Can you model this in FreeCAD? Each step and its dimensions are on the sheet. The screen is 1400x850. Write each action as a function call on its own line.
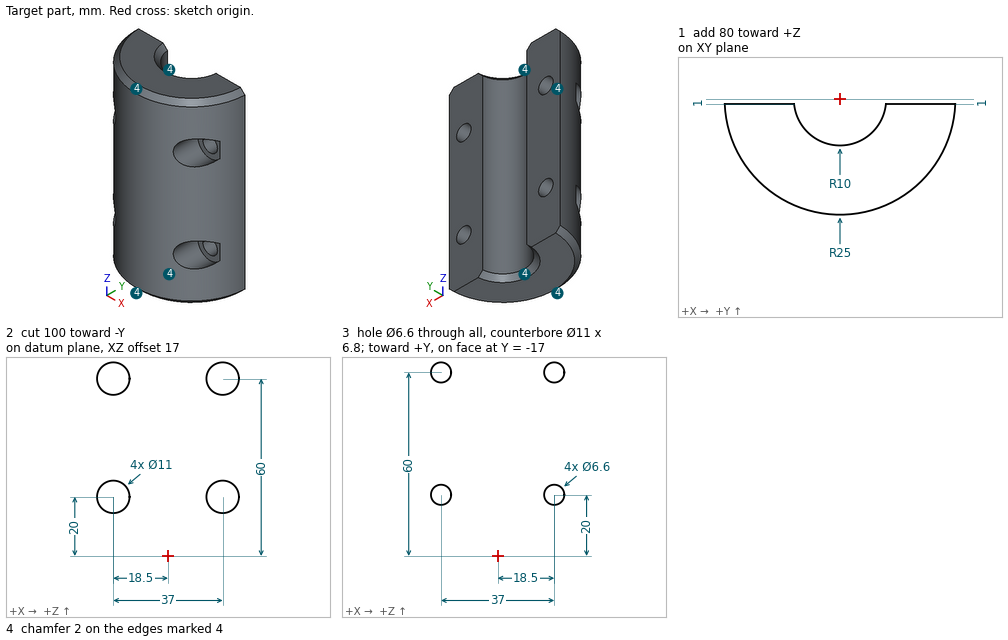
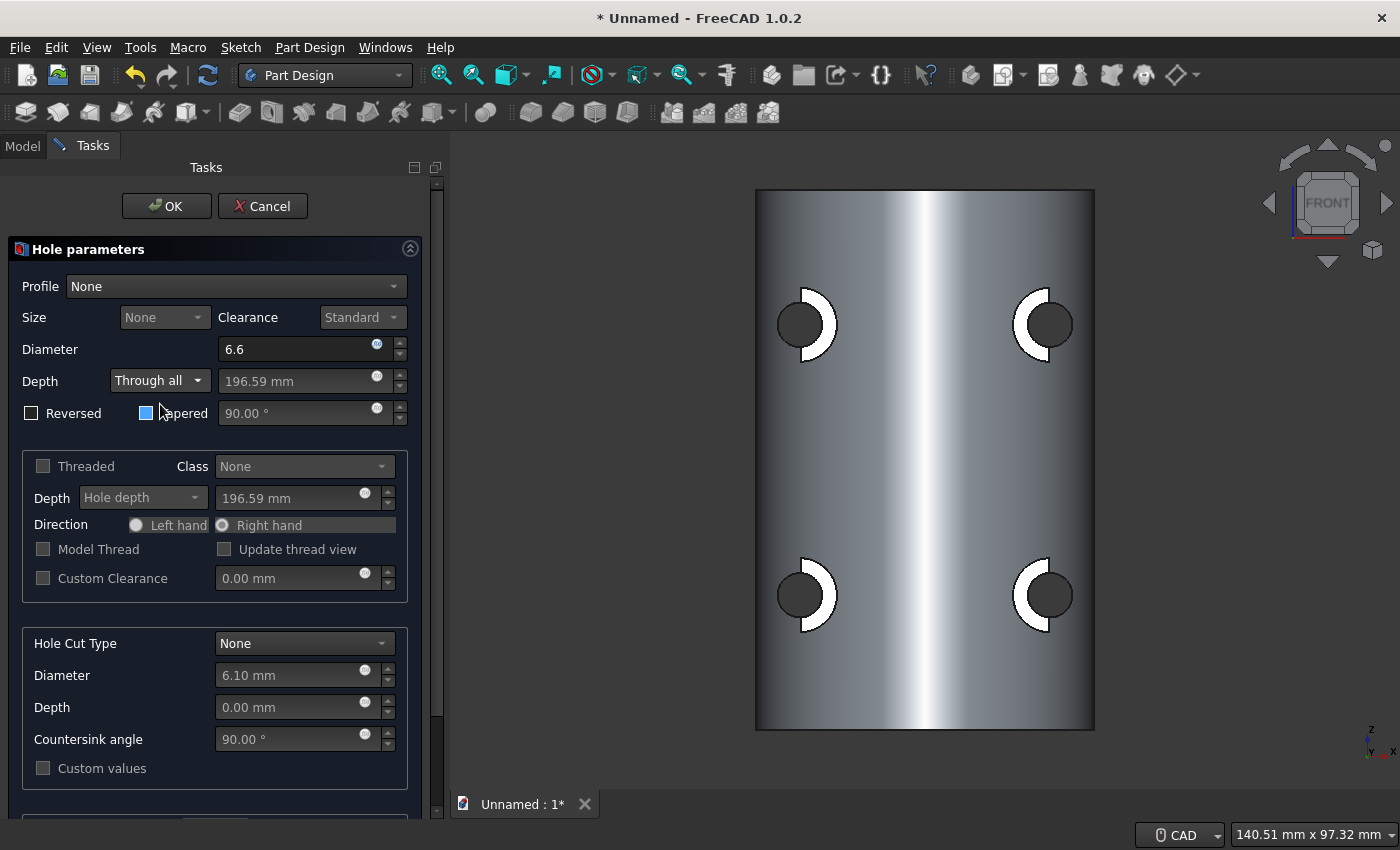
click(306, 644)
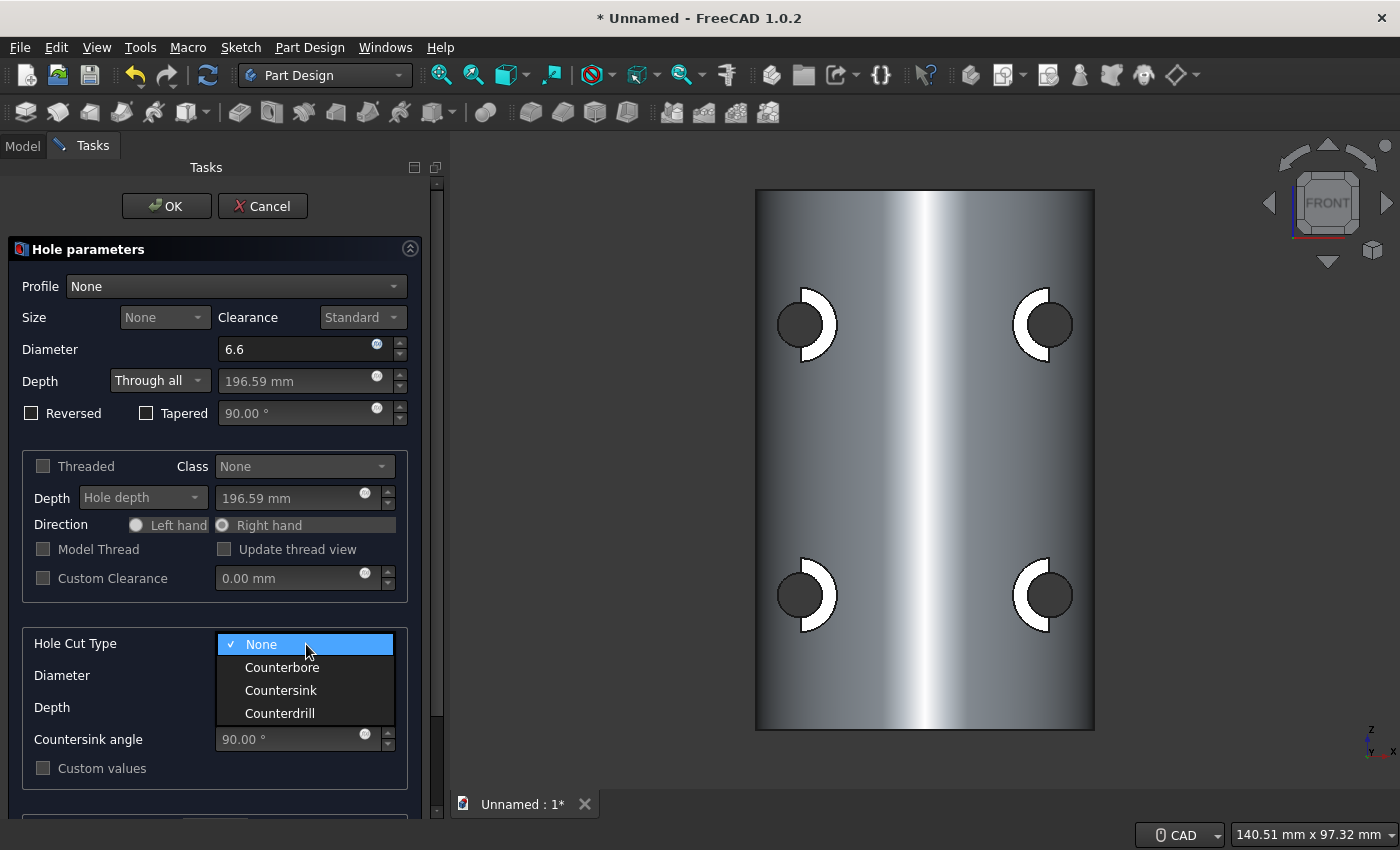
click(304, 668)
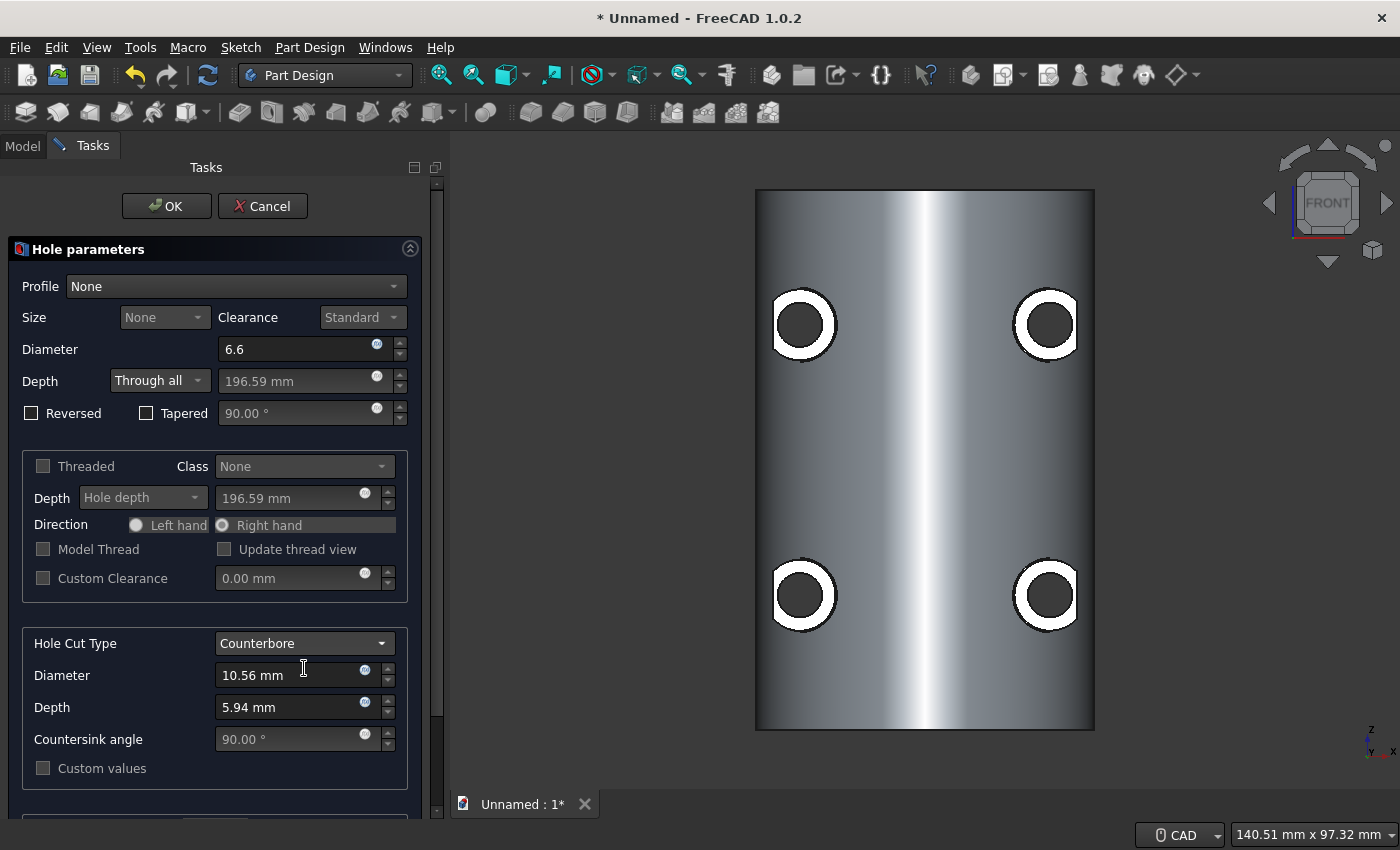
triple_click(298, 675)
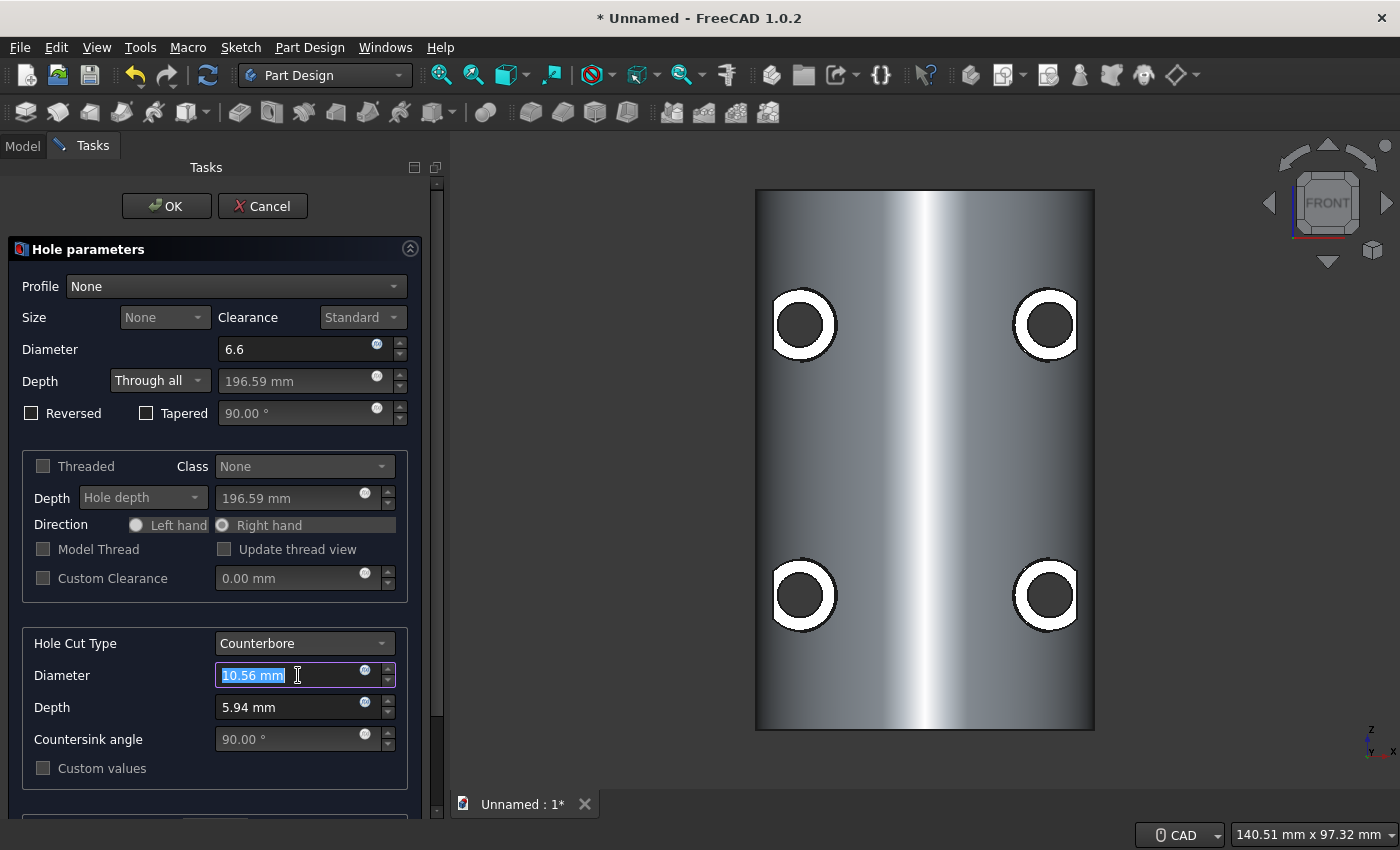
text(11)
key(Tab)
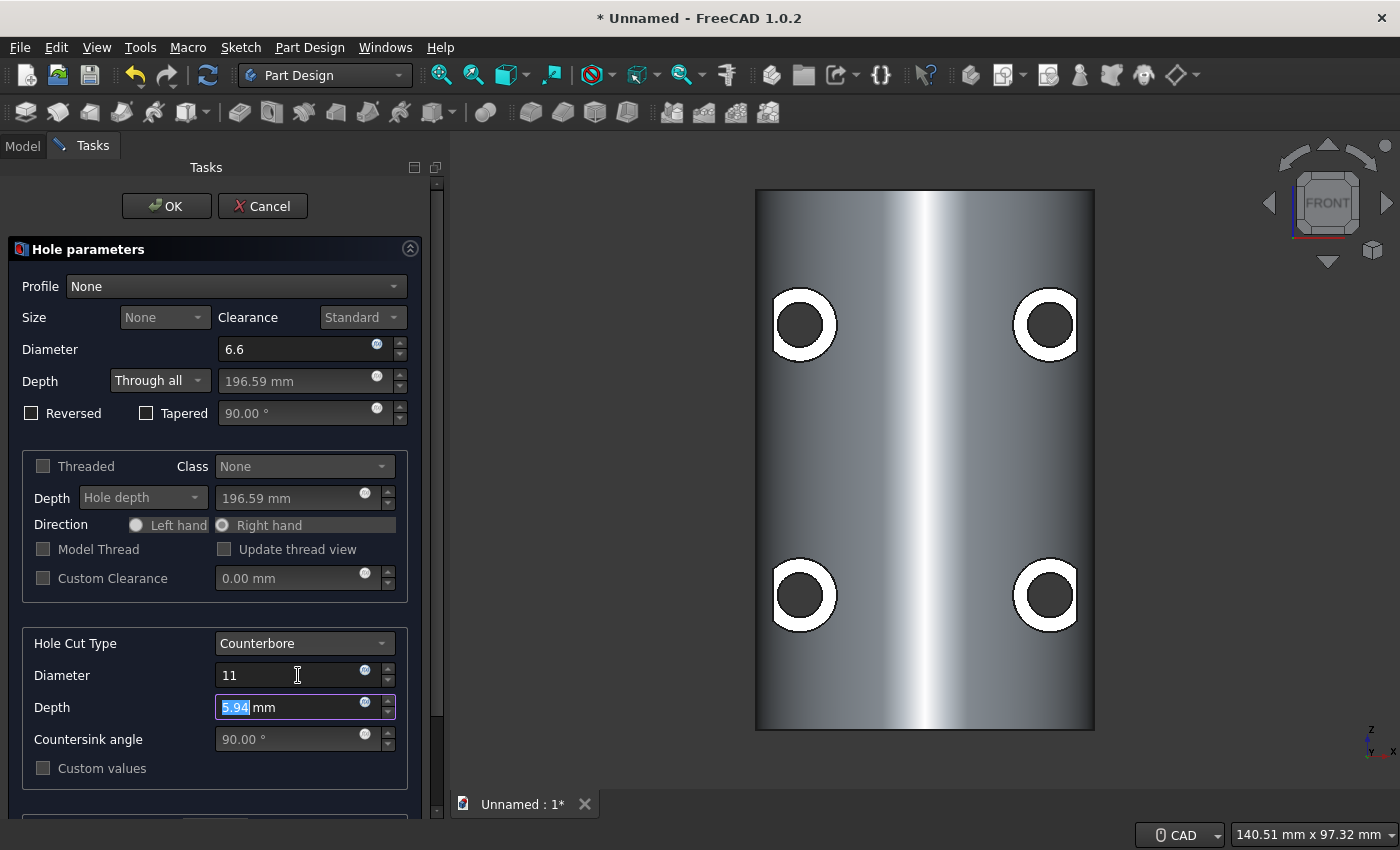
text(6.8)
key(Tab)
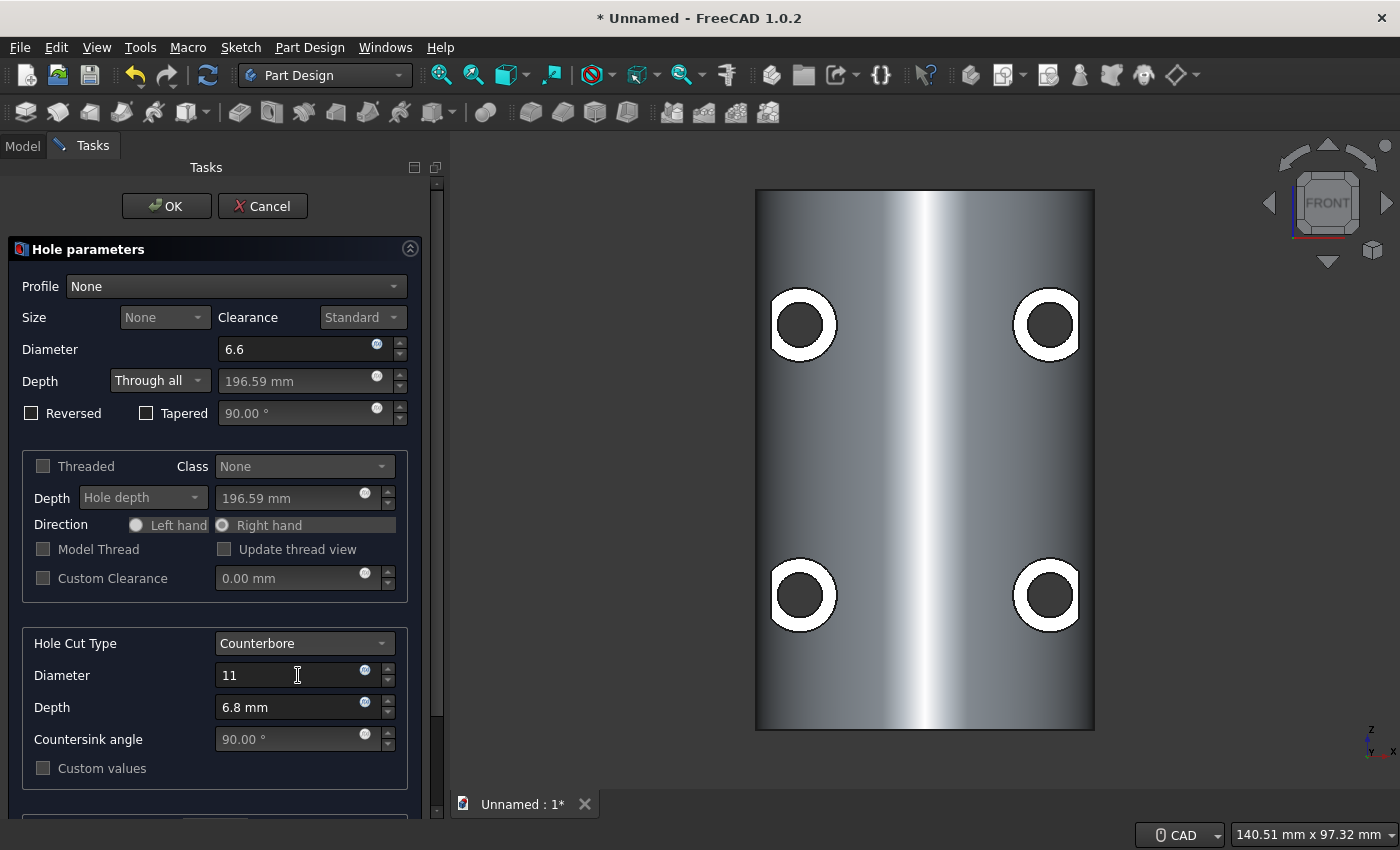
click(167, 206)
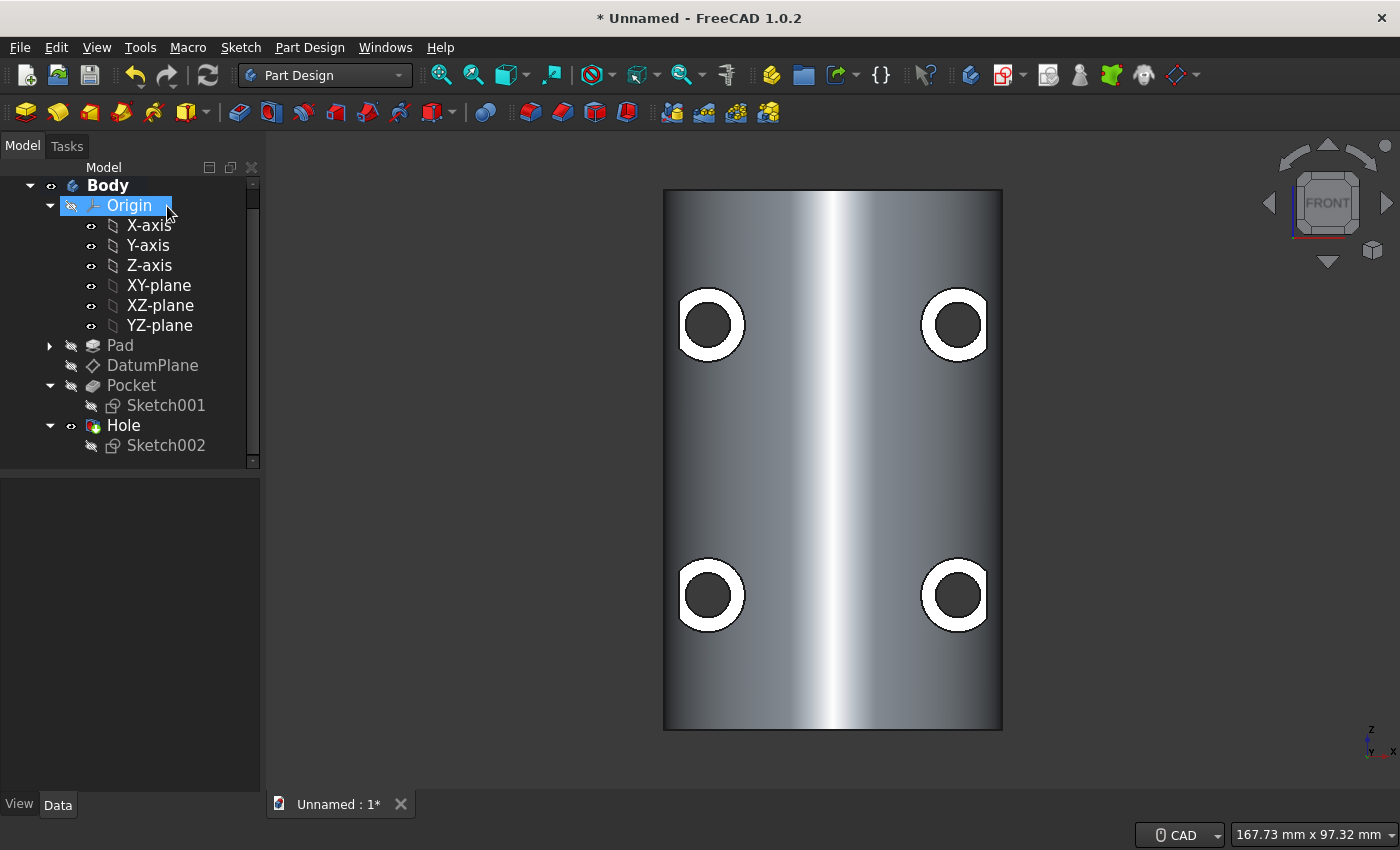
click(833, 189)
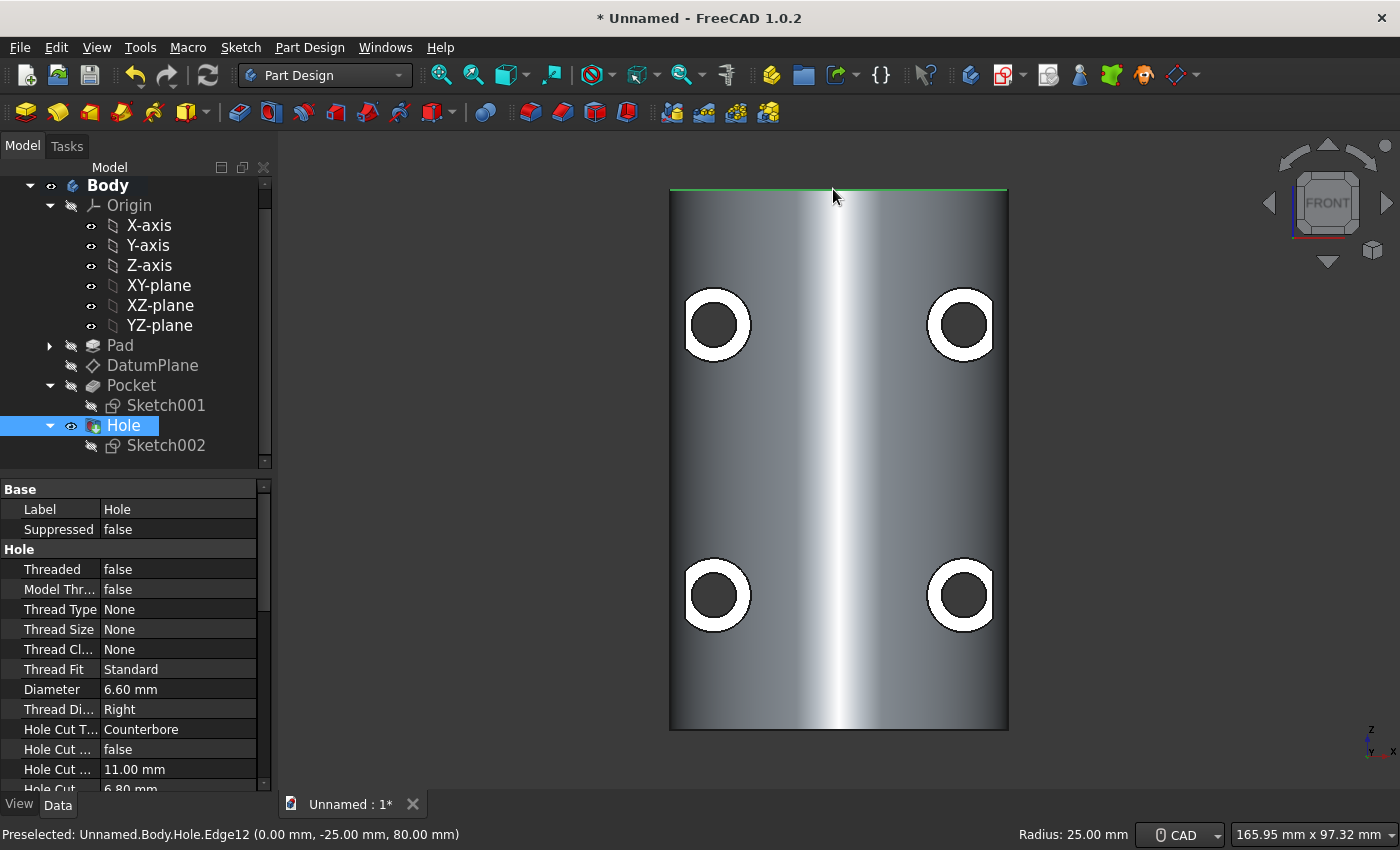
click(839, 729, ctrl)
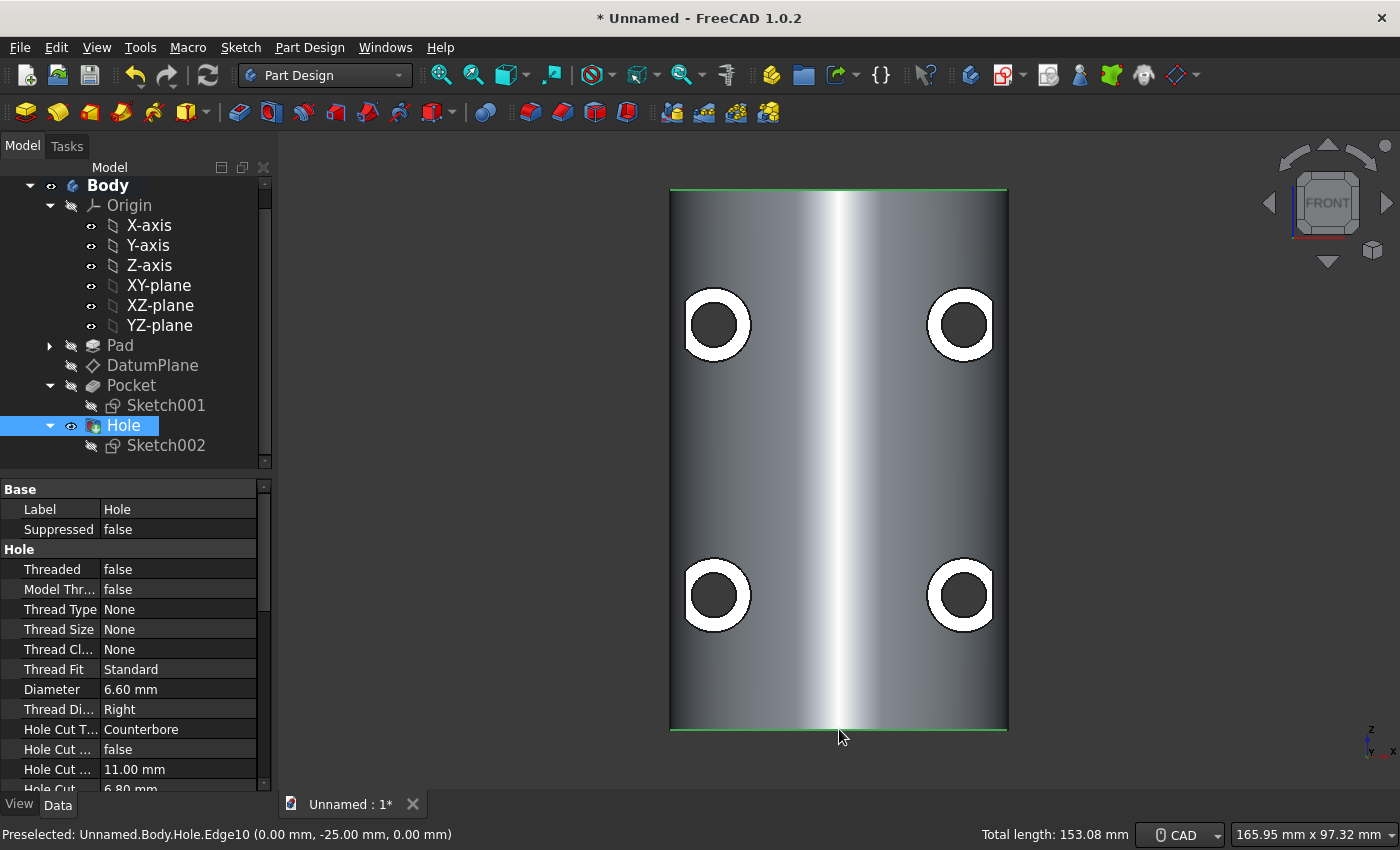
key(0)